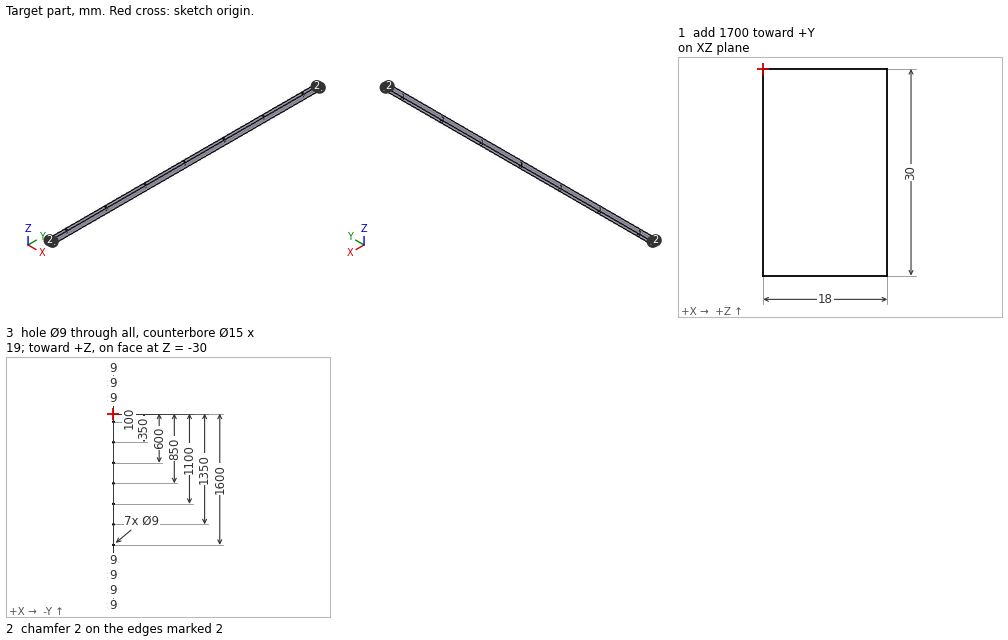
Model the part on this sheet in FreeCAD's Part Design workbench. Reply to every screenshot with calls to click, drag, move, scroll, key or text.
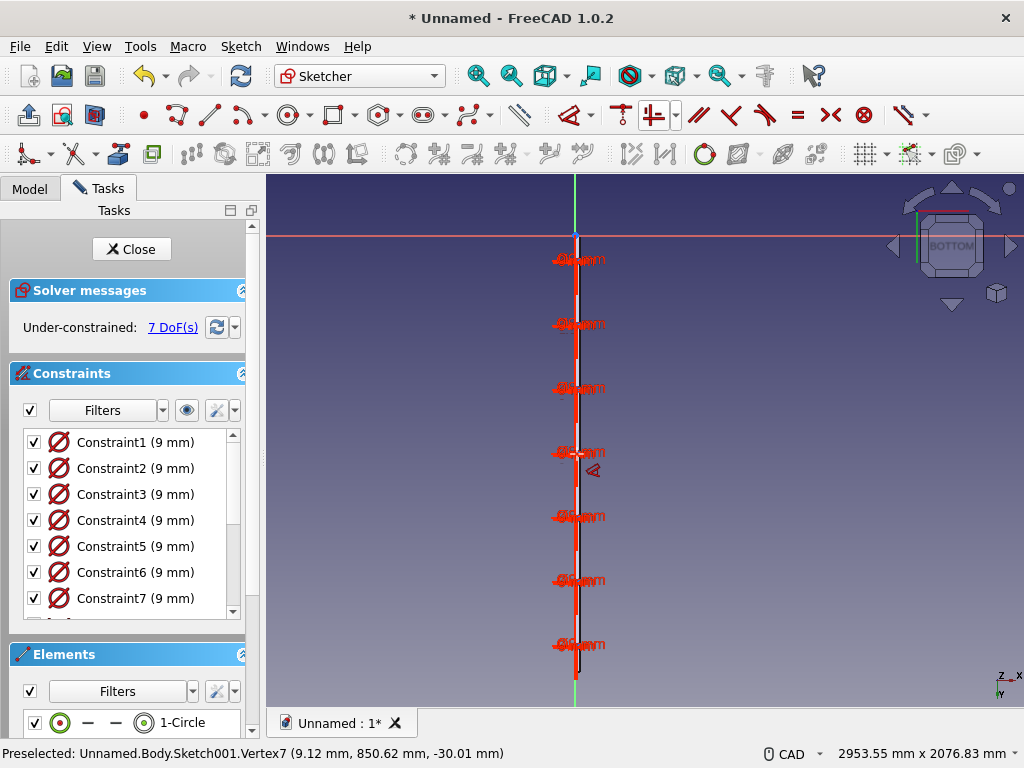
click(577, 390)
click(541, 348)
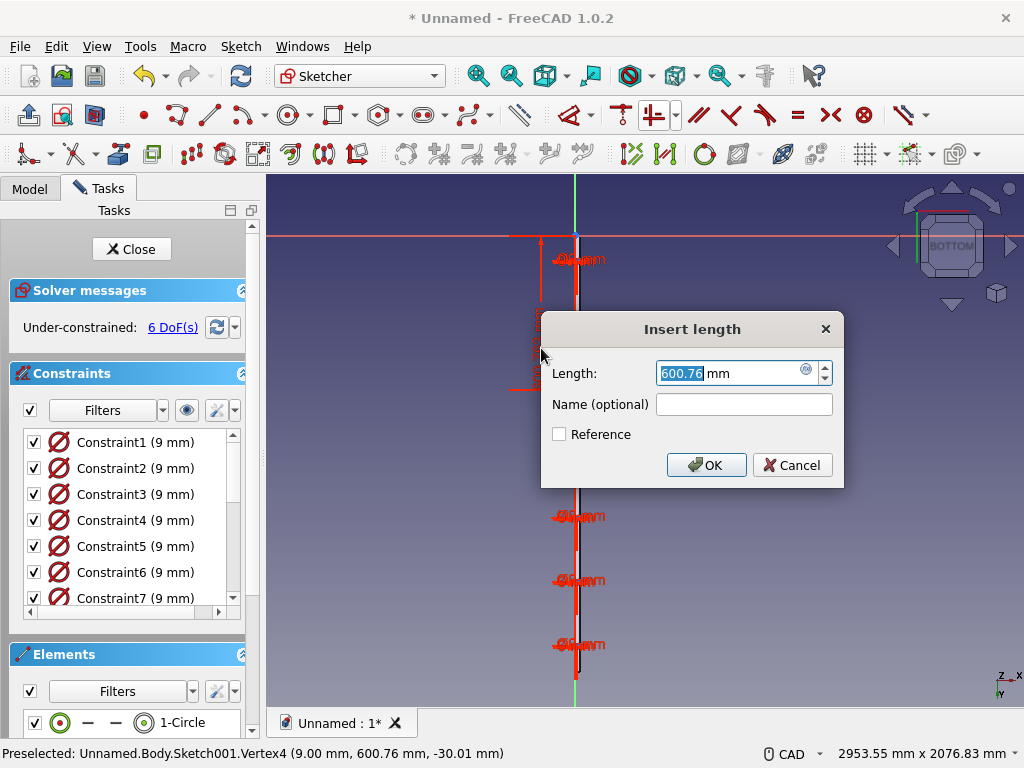
text(600)
key(Return)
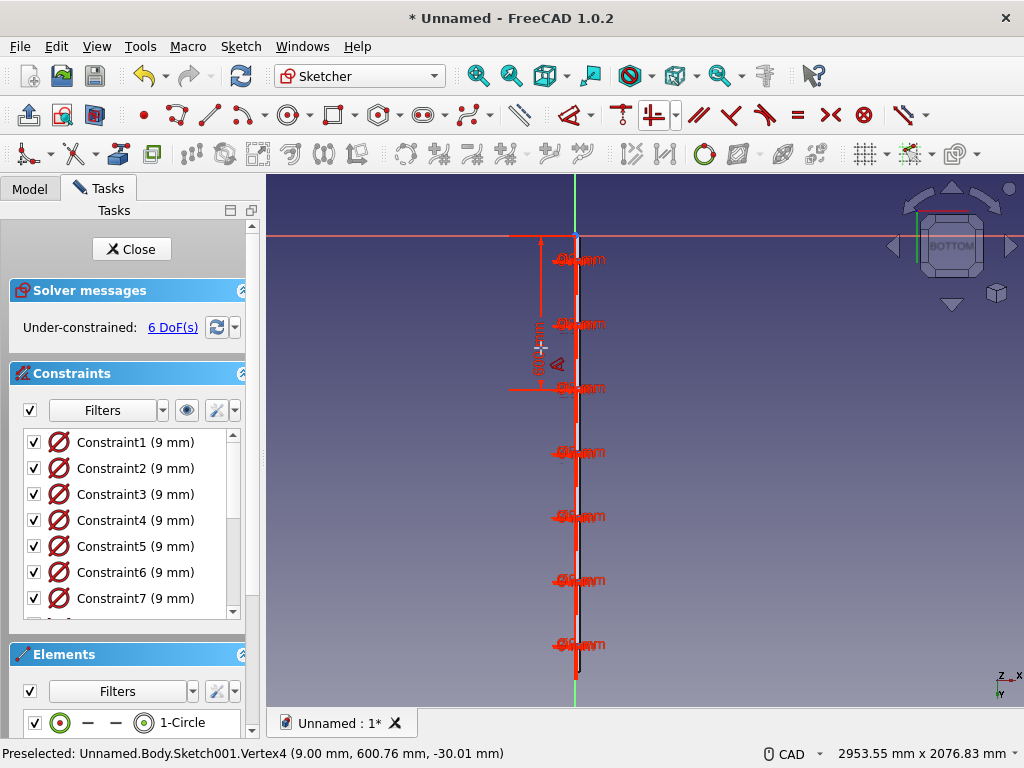
click(577, 326)
click(541, 301)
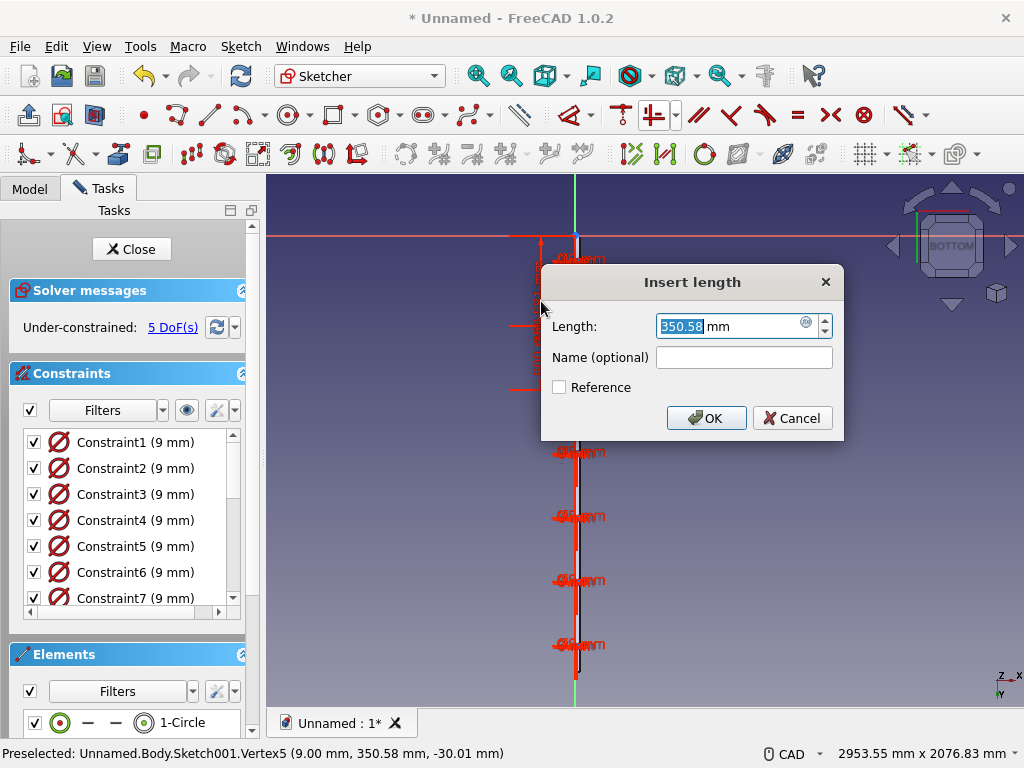
text(350)
key(Return)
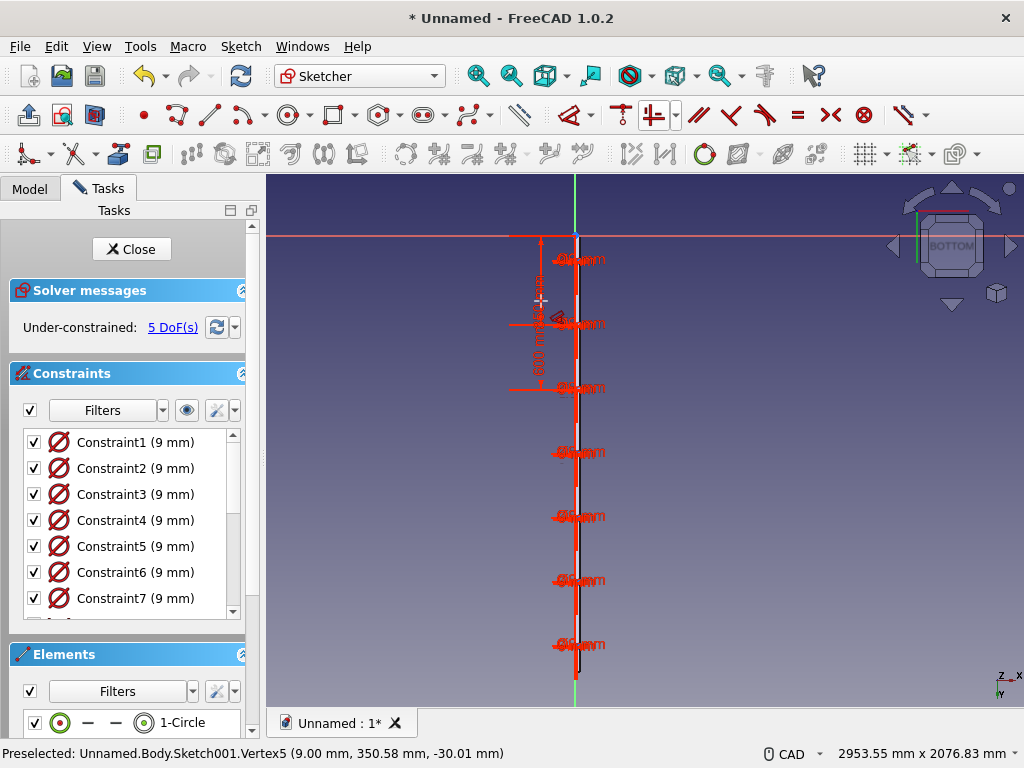
scroll(577, 261, up, 3)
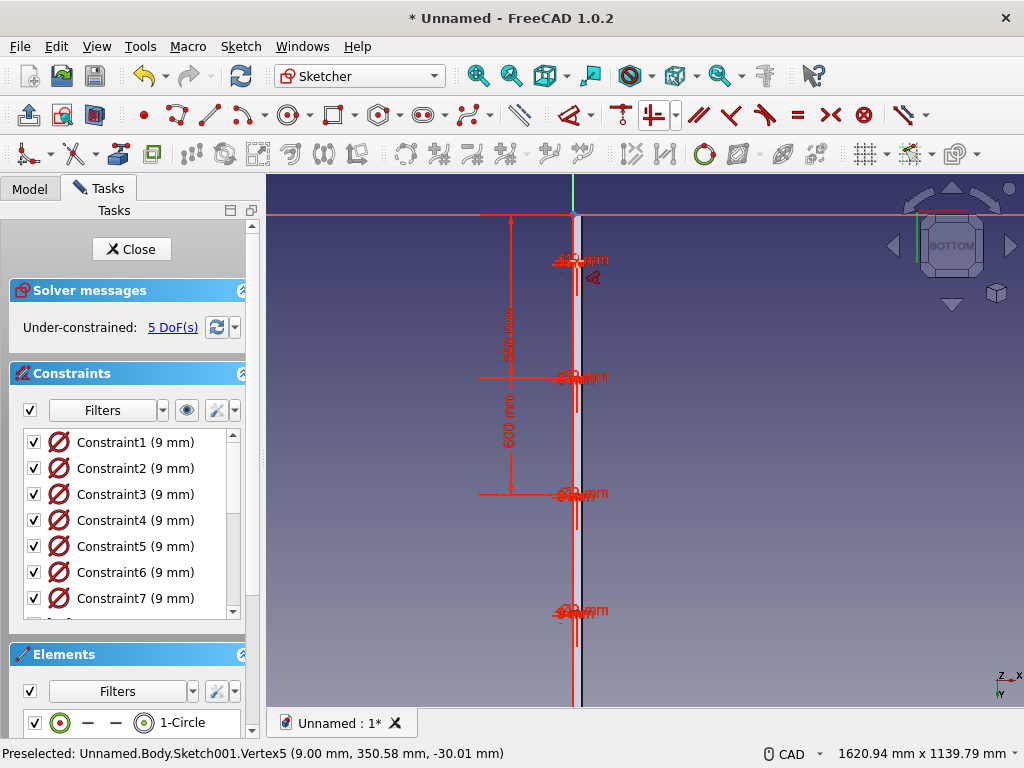
click(577, 261)
click(539, 238)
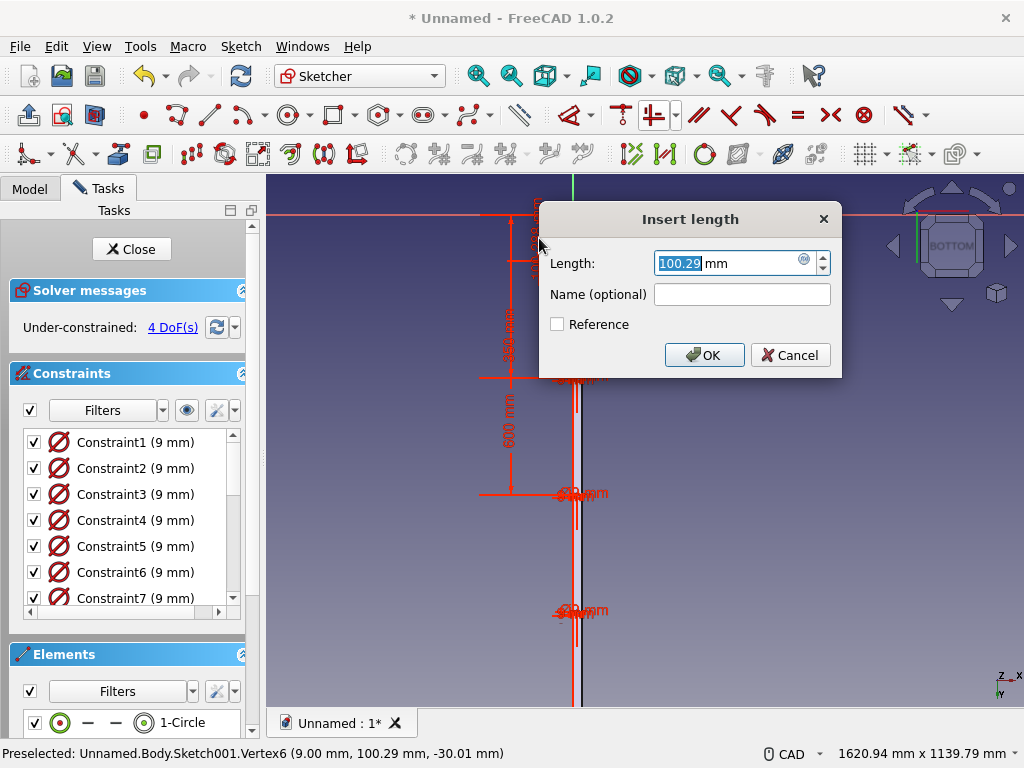
text(100)
key(Return)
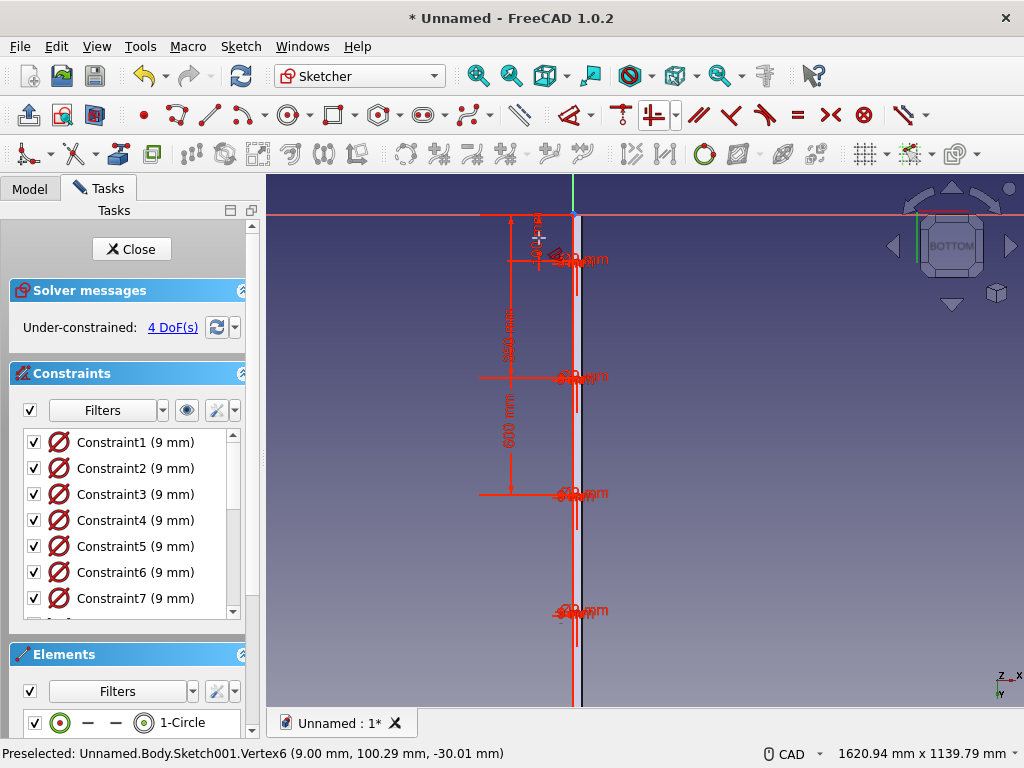
click(577, 612)
click(539, 553)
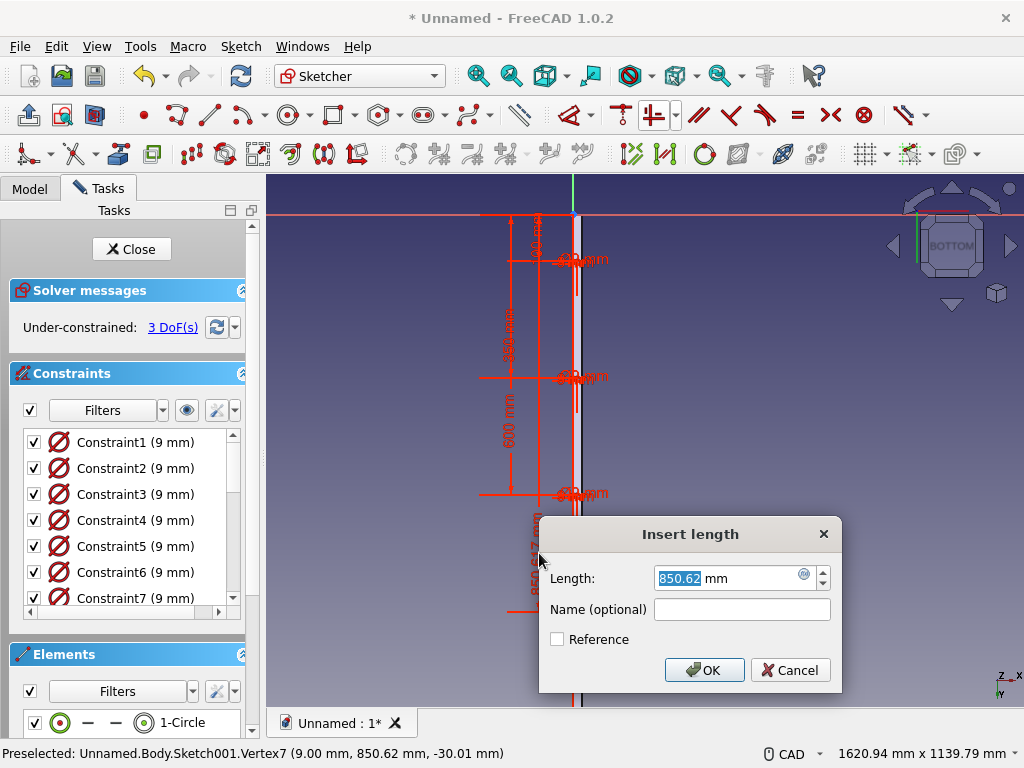
text(850)
key(Return)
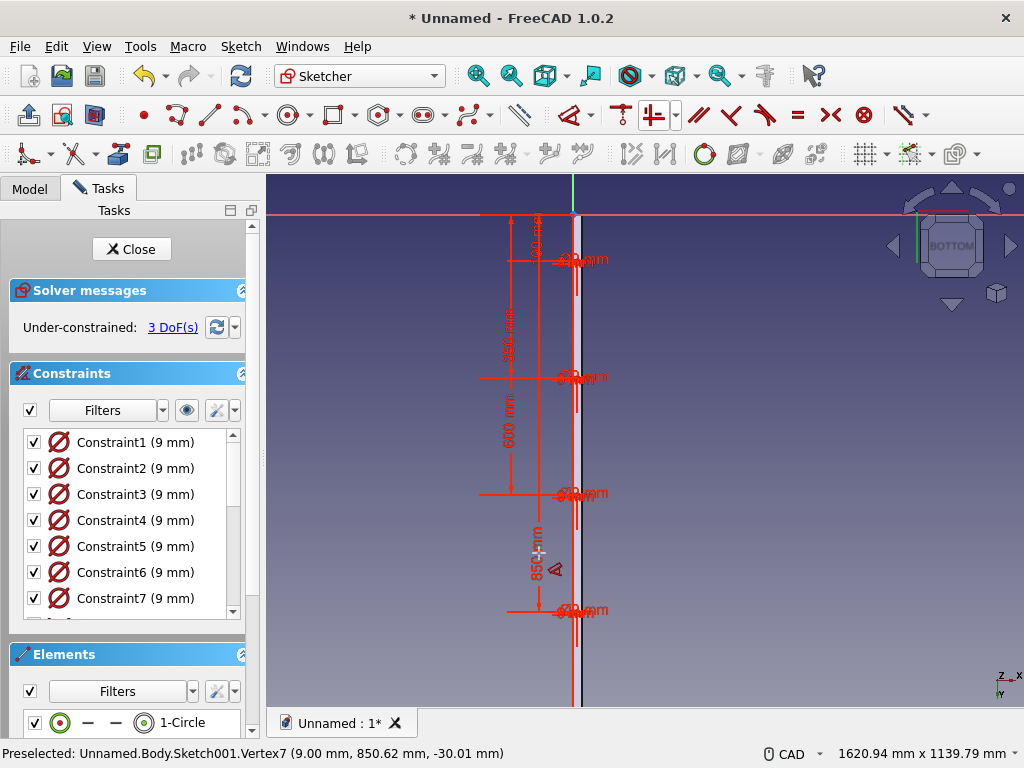
scroll(577, 319, down, 4)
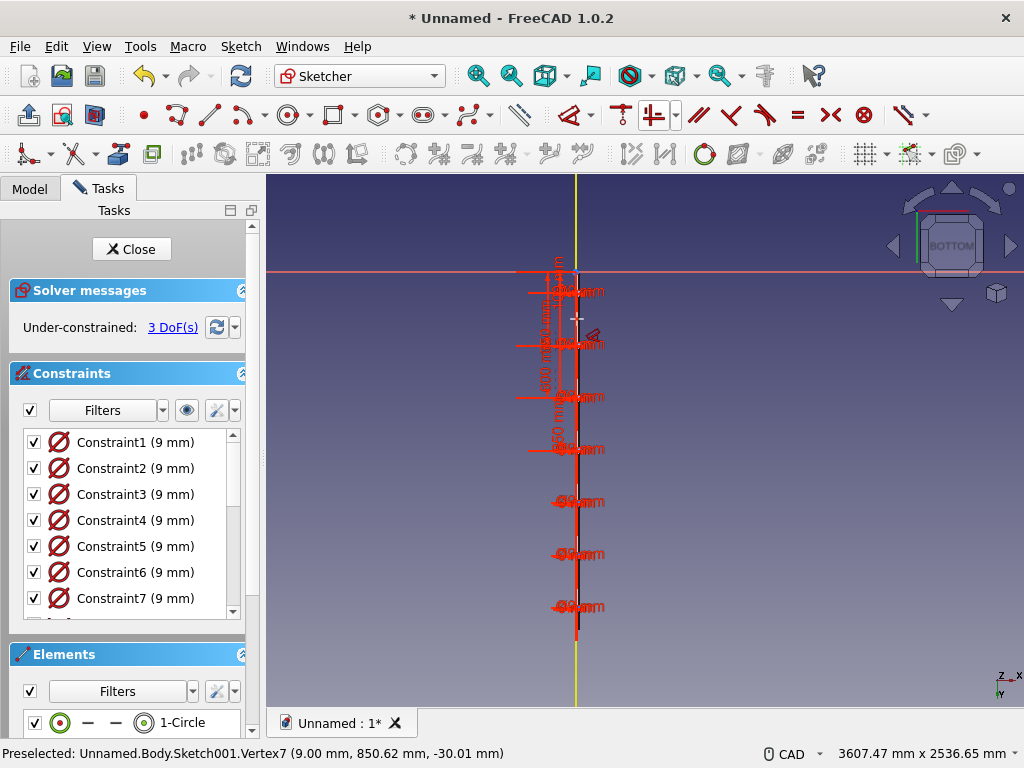
click(577, 608)
click(635, 323)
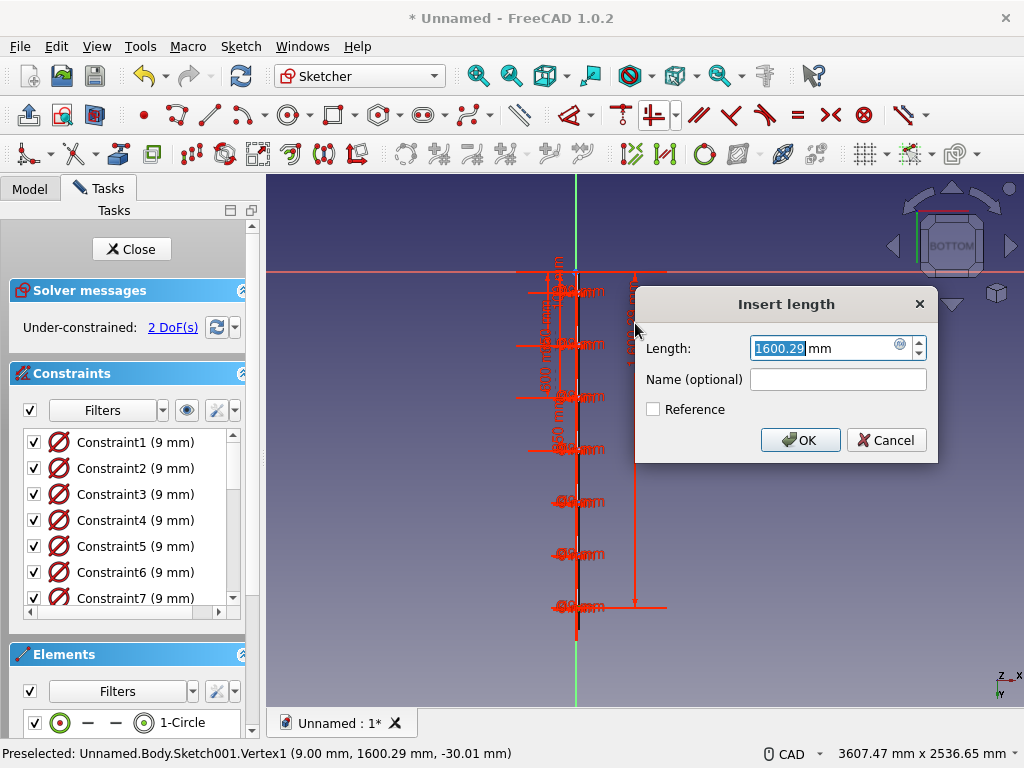
text(1600)
key(Return)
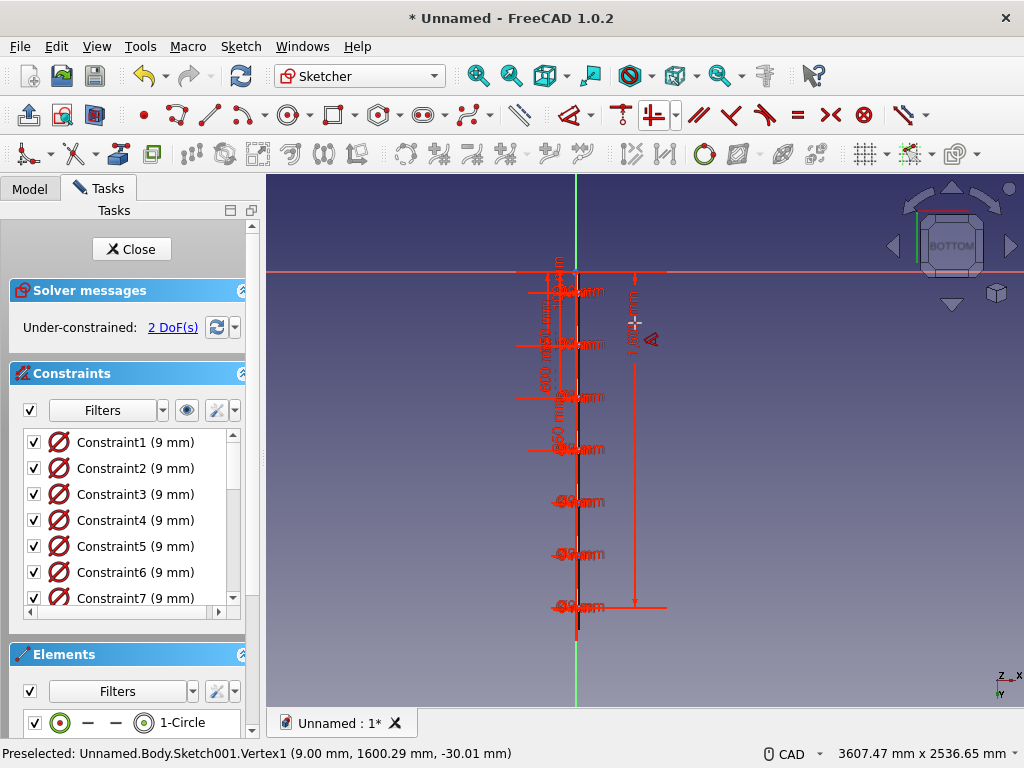
click(577, 556)
click(542, 479)